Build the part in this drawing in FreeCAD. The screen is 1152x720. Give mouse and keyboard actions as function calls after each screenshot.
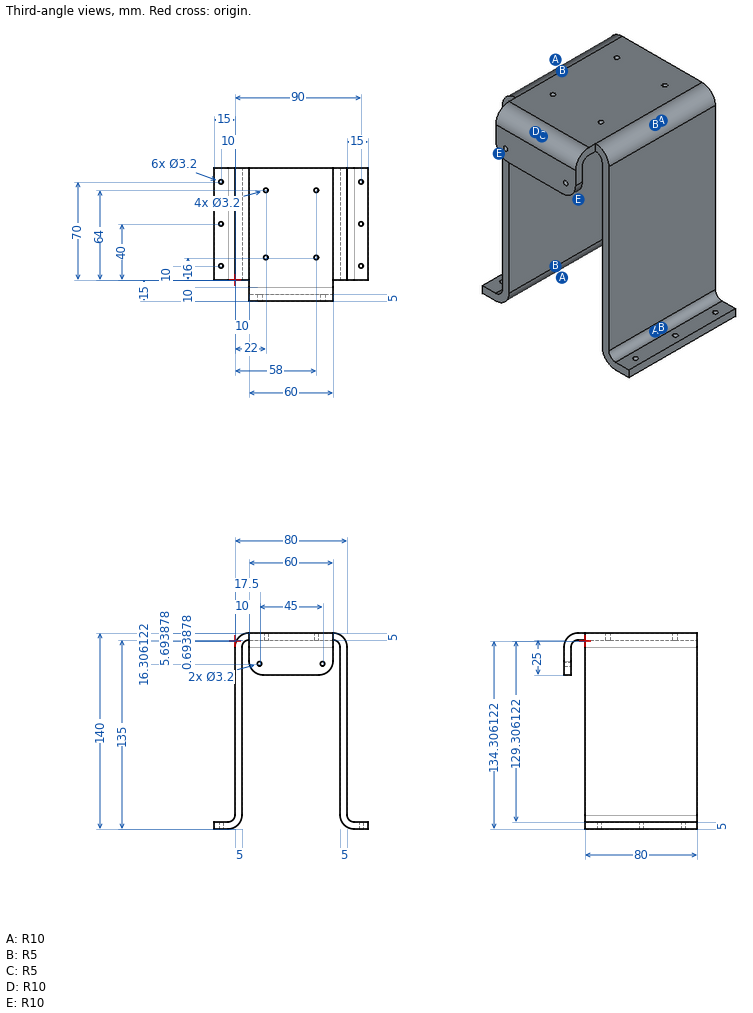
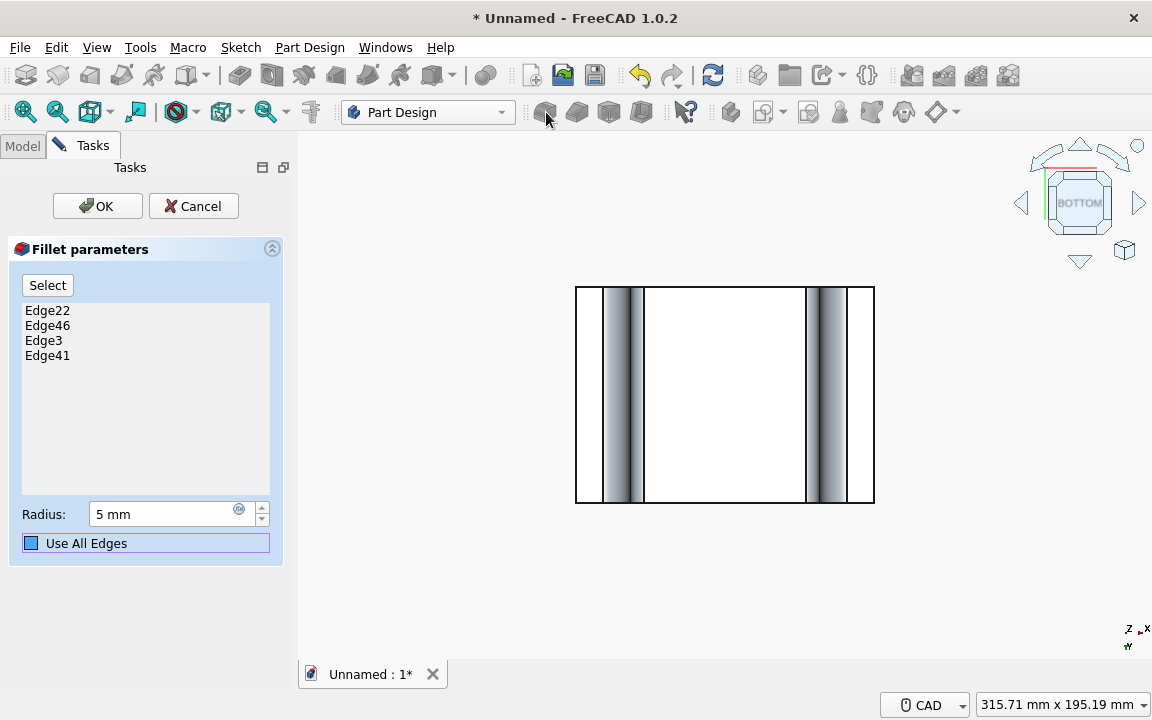
click(98, 206)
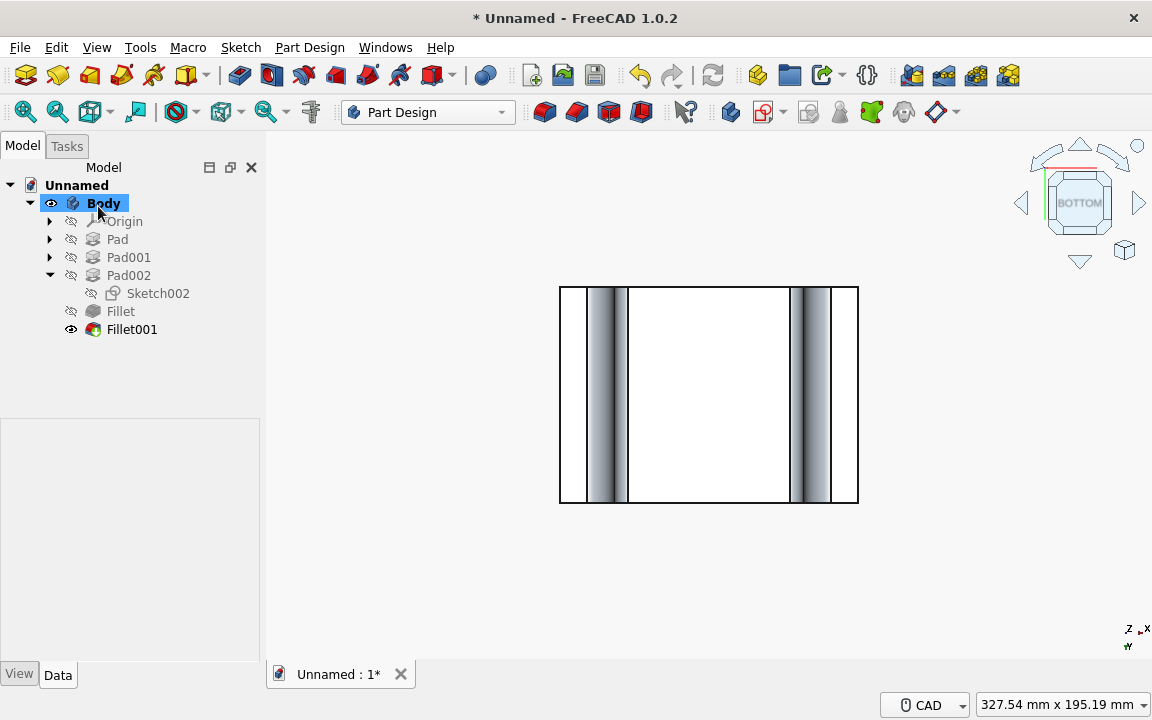
click(26, 112)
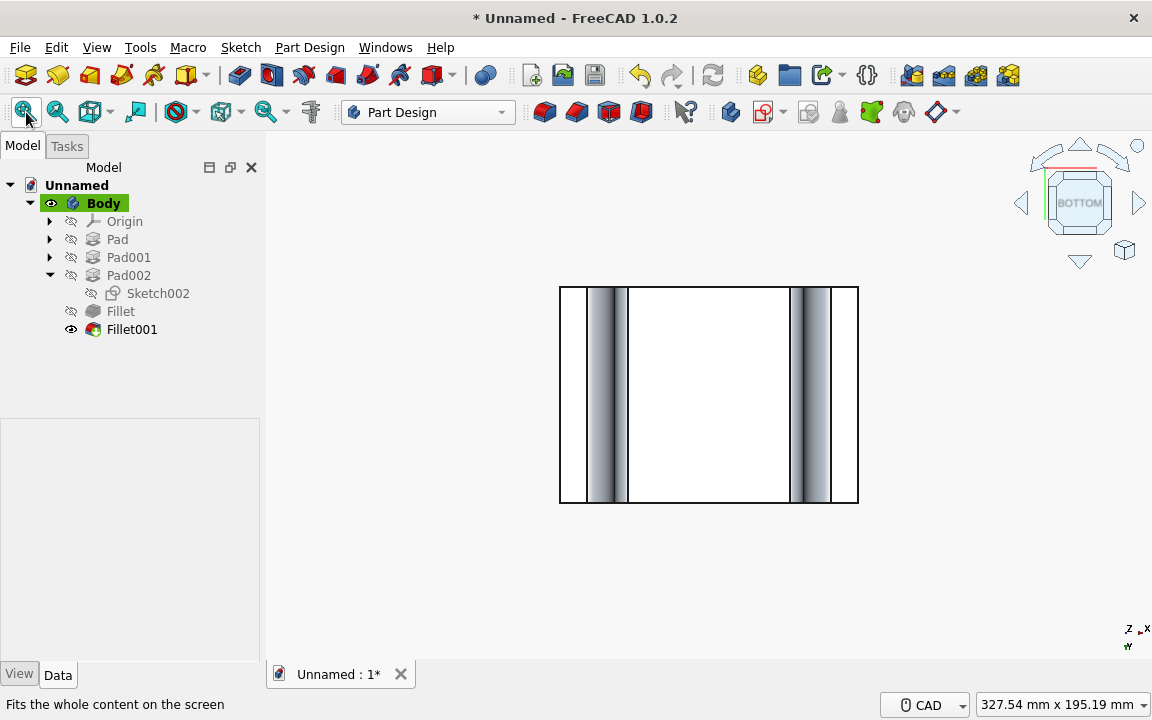
click(764, 112)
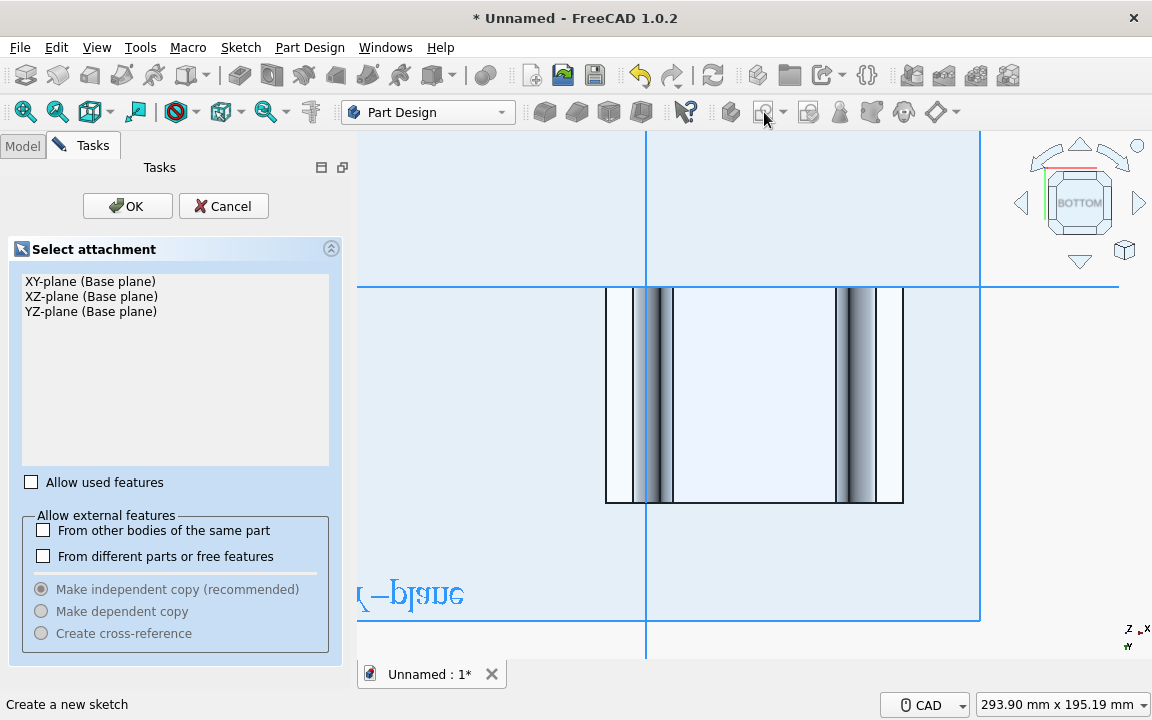
click(82, 296)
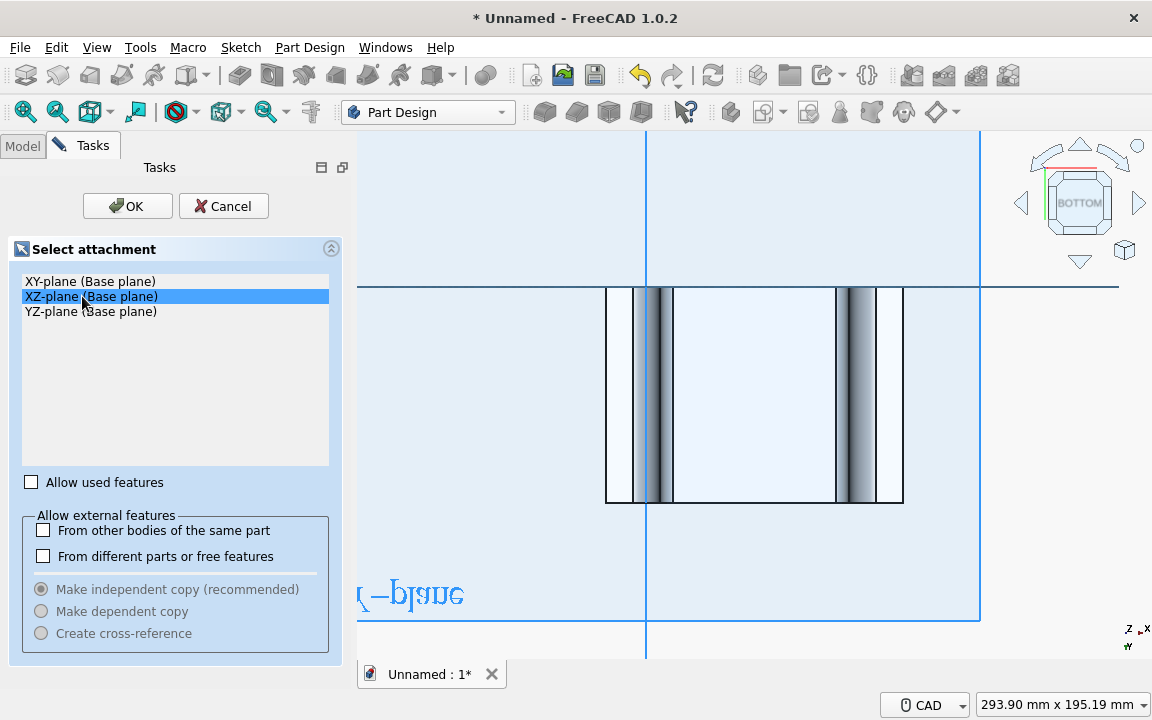
click(128, 206)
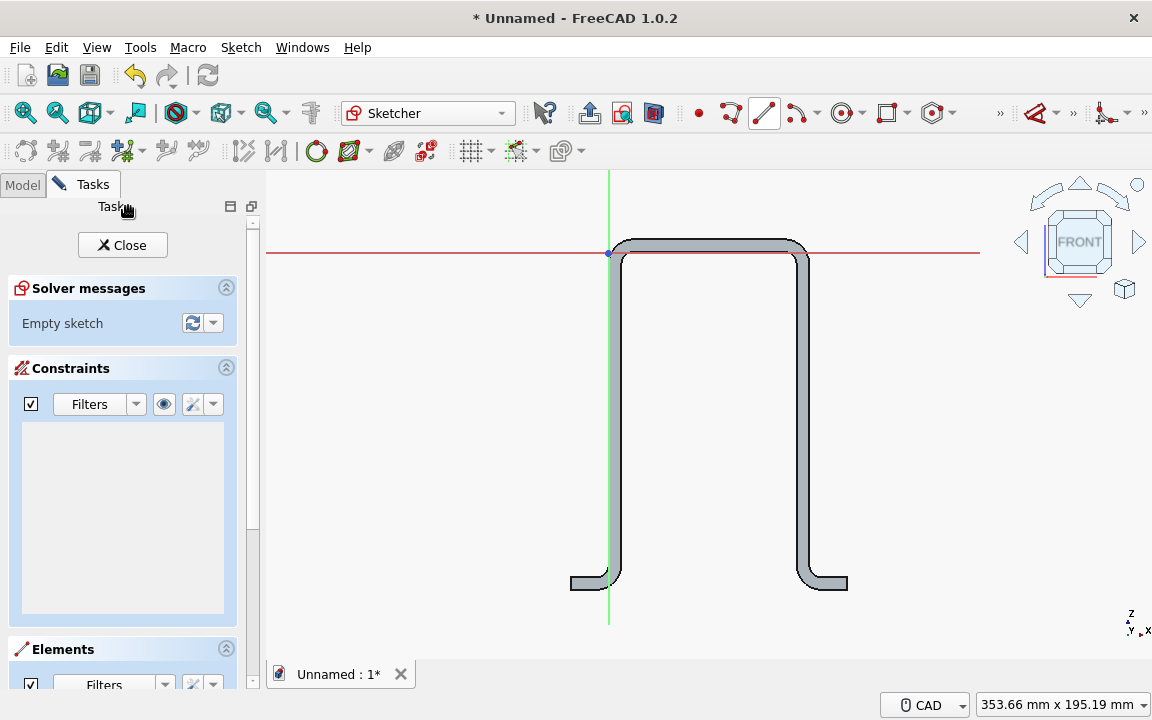
scroll(729, 198, up, 5)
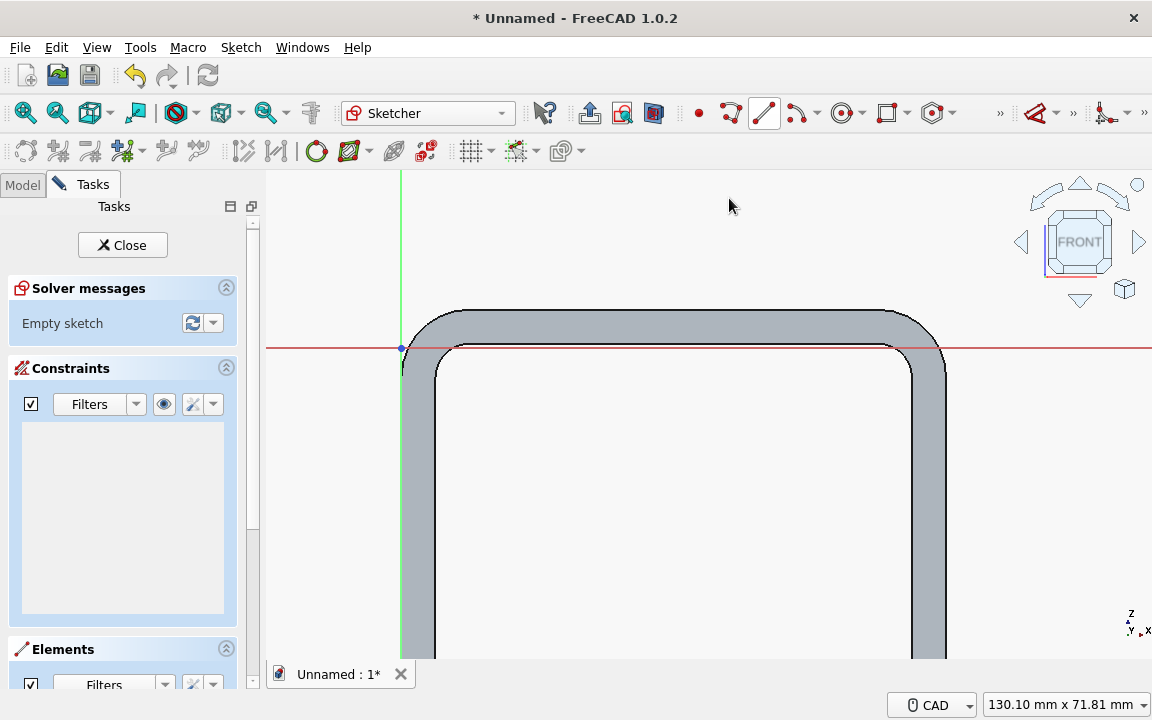
click(888, 114)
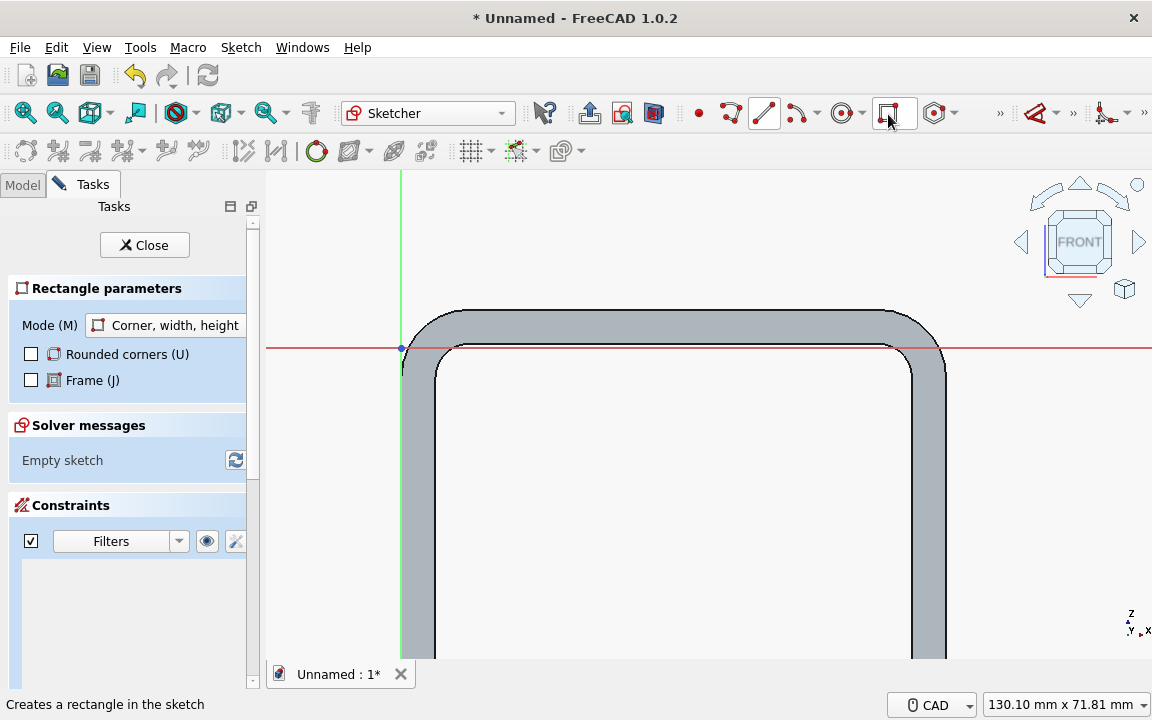
click(469, 310)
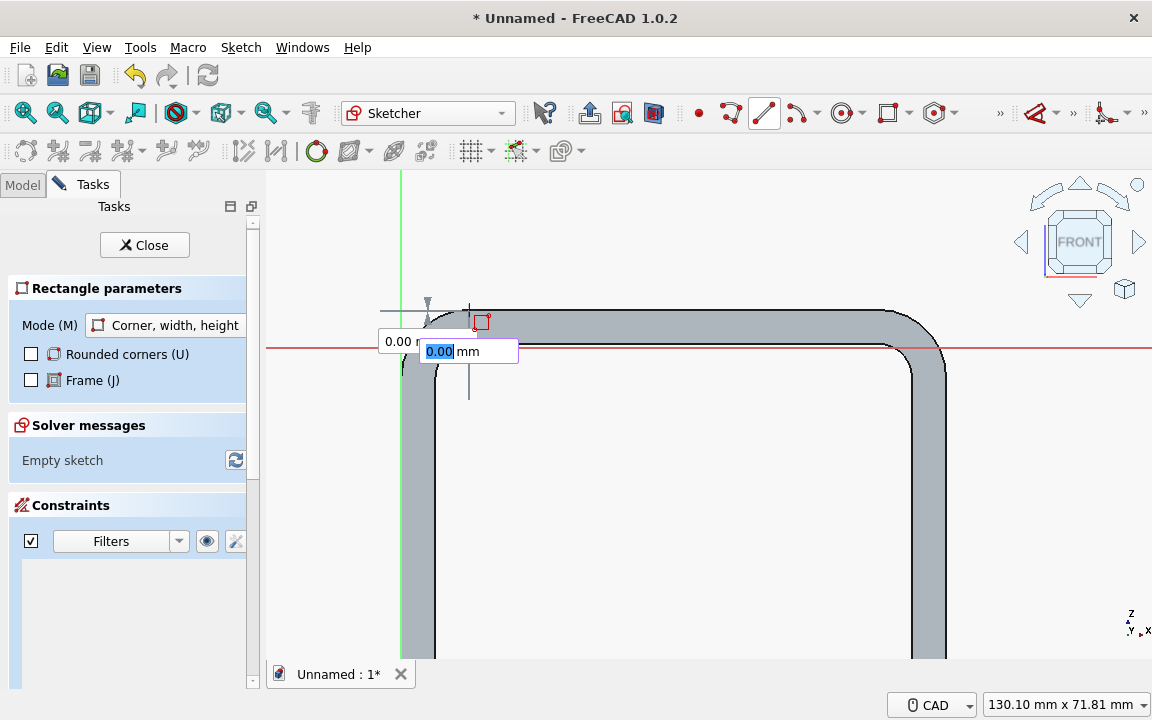
scroll(878, 344, up, 7)
move(876, 342)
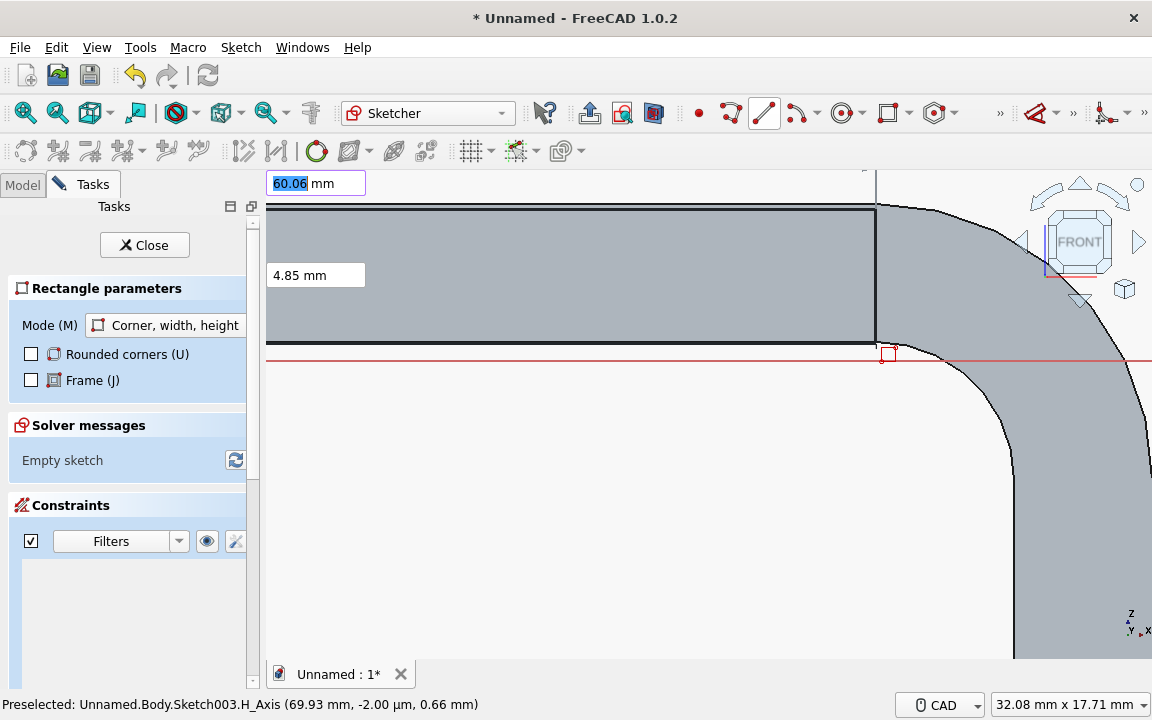
text(60)
key(Tab)
text(5)
key(Return)
key(Escape)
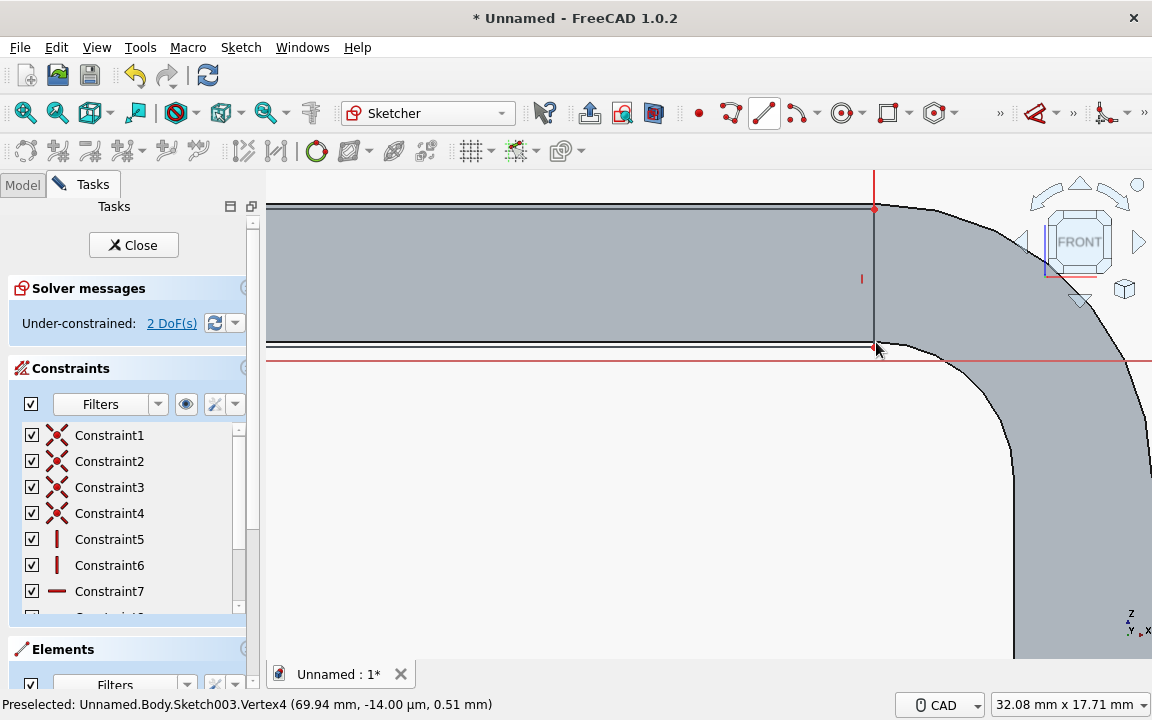
click(1036, 114)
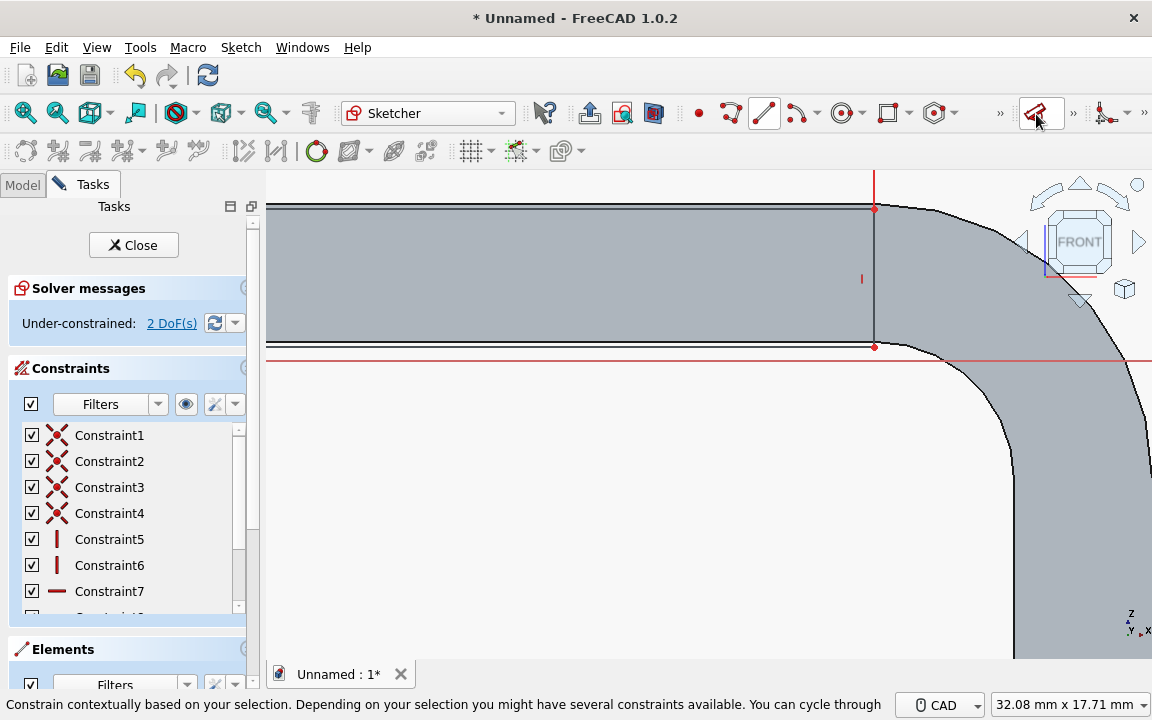
scroll(880, 458, down, 7)